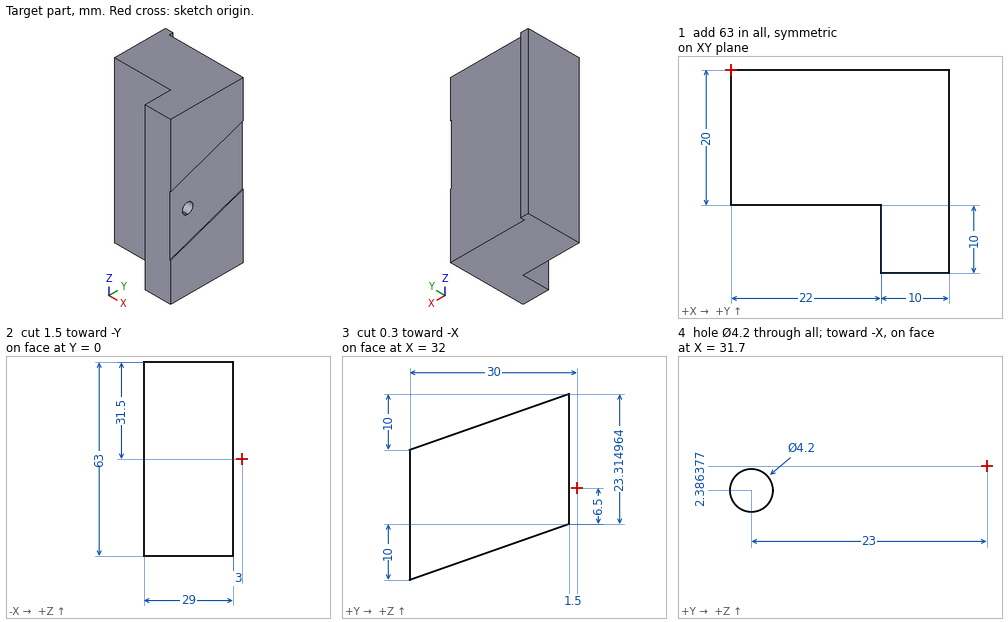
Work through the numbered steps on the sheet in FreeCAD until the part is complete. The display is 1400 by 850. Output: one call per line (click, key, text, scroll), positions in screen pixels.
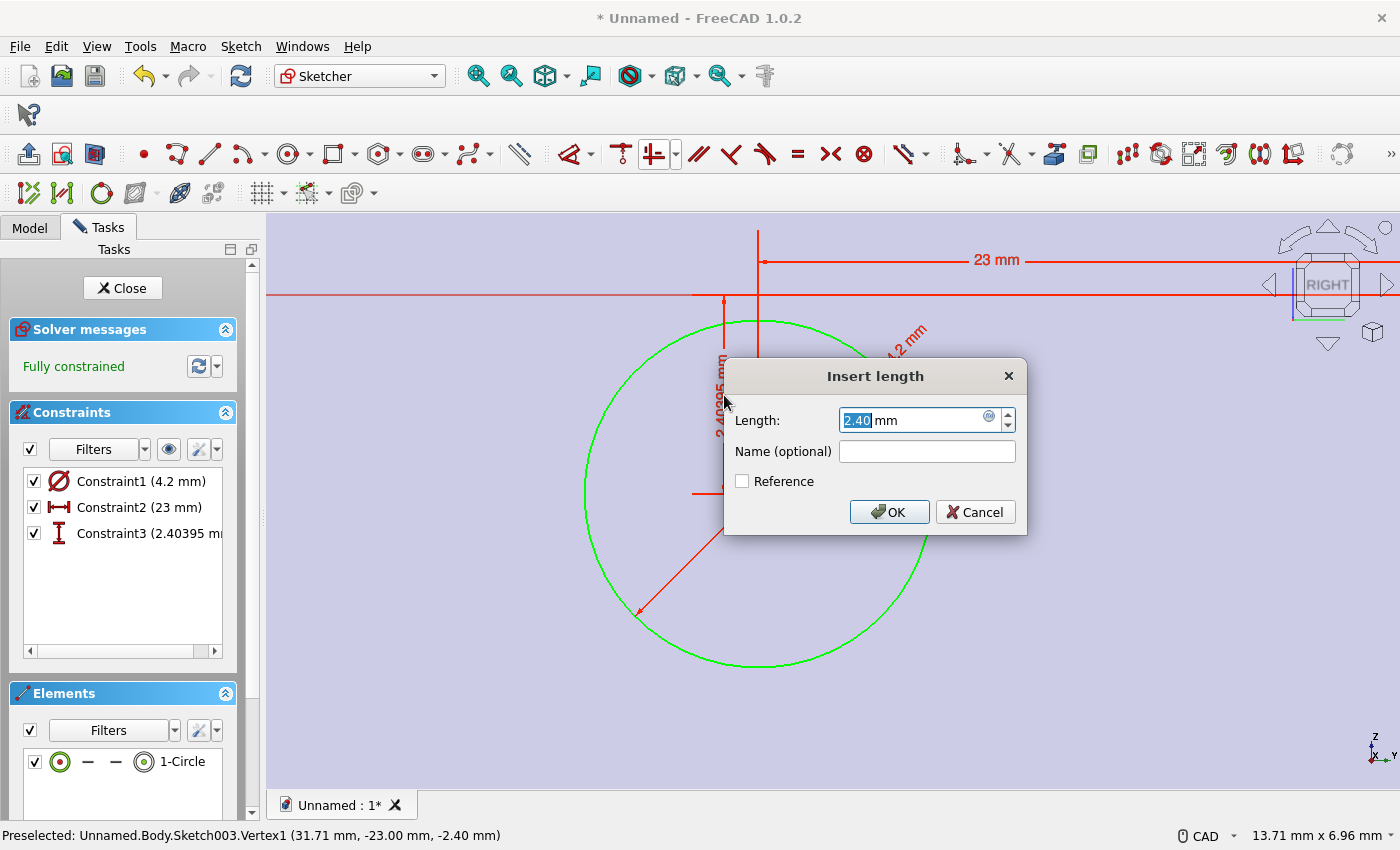
text(2.386377)
key(Return)
key(Escape)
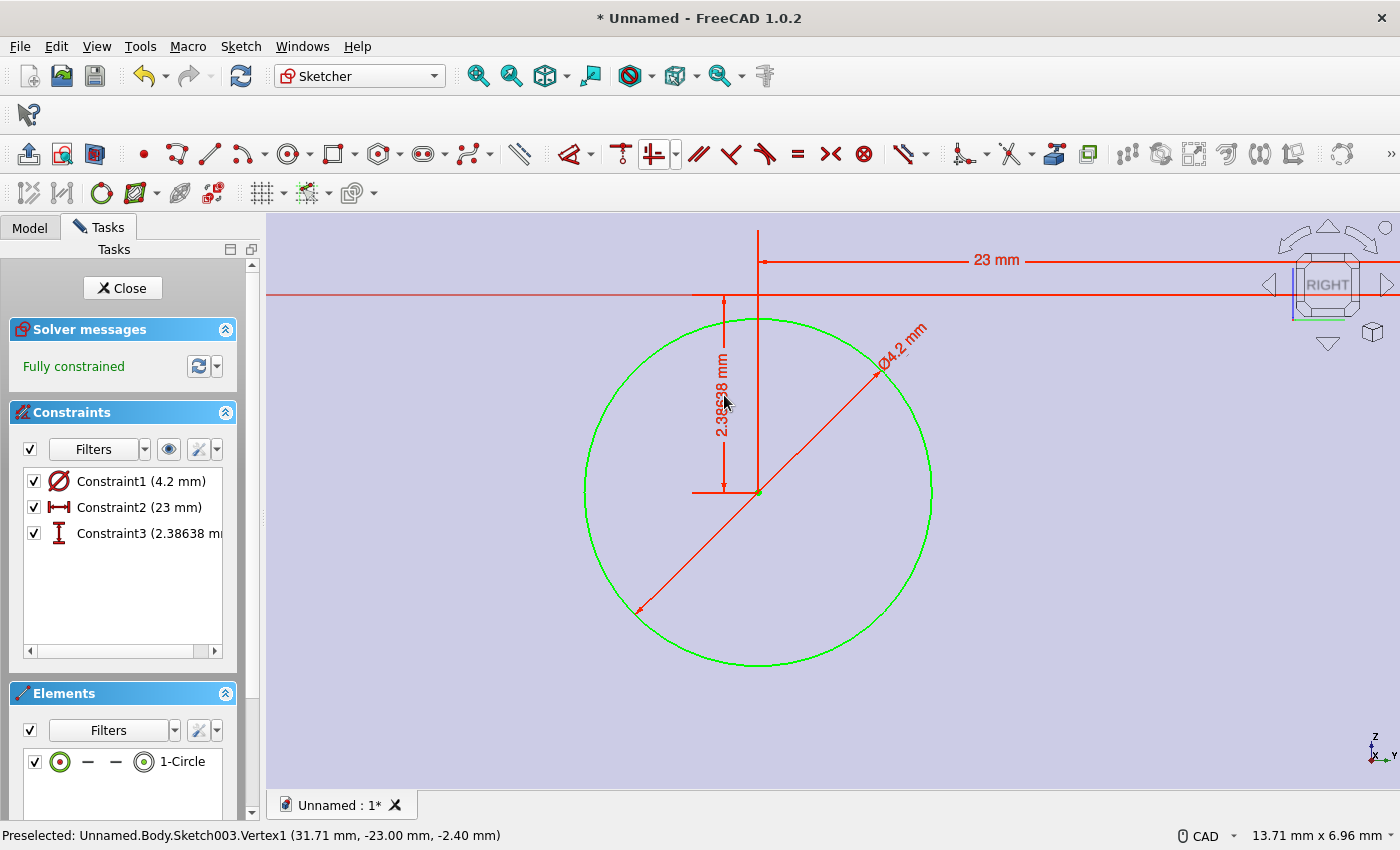
click(123, 288)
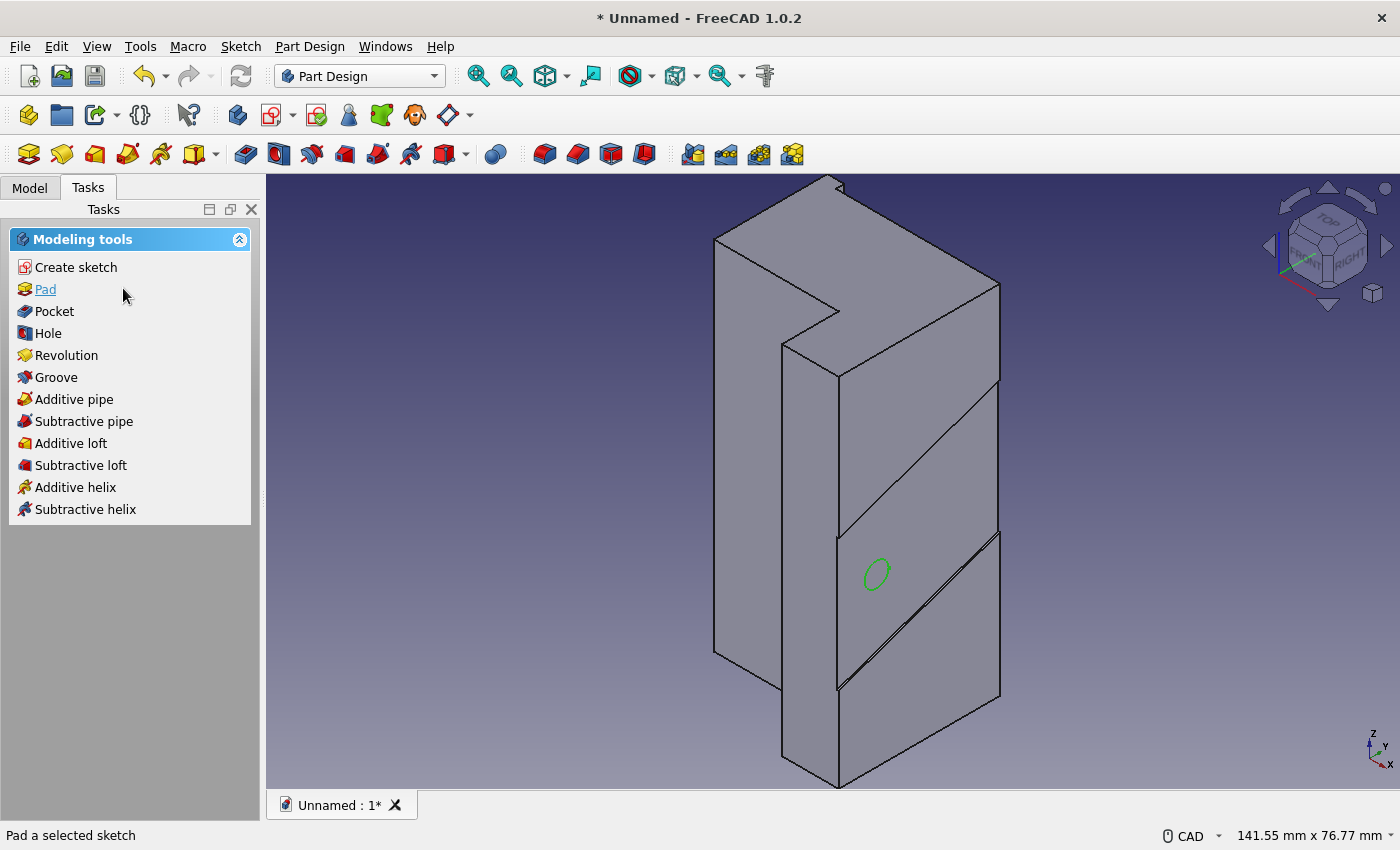
click(279, 154)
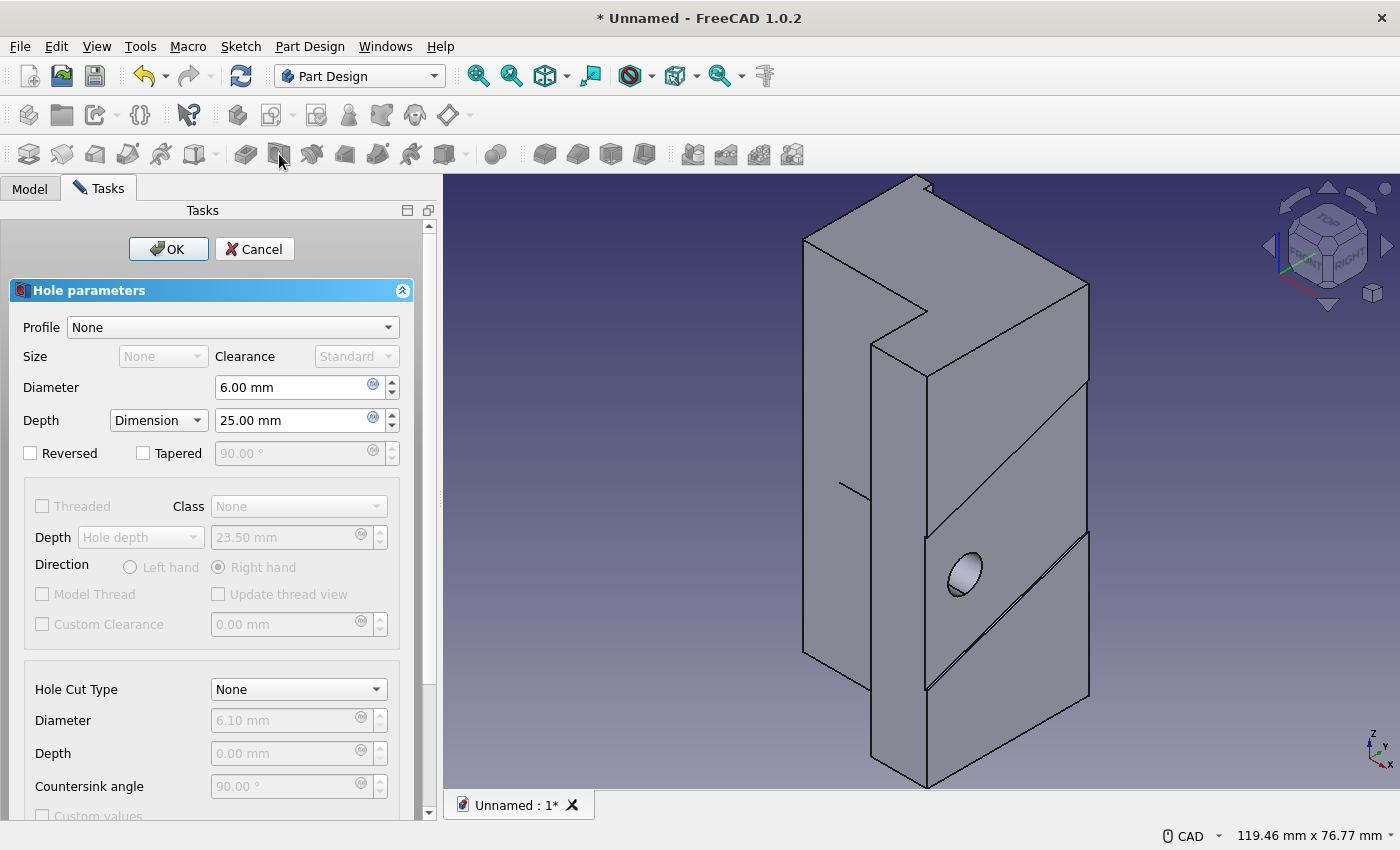
triple_click(300, 388)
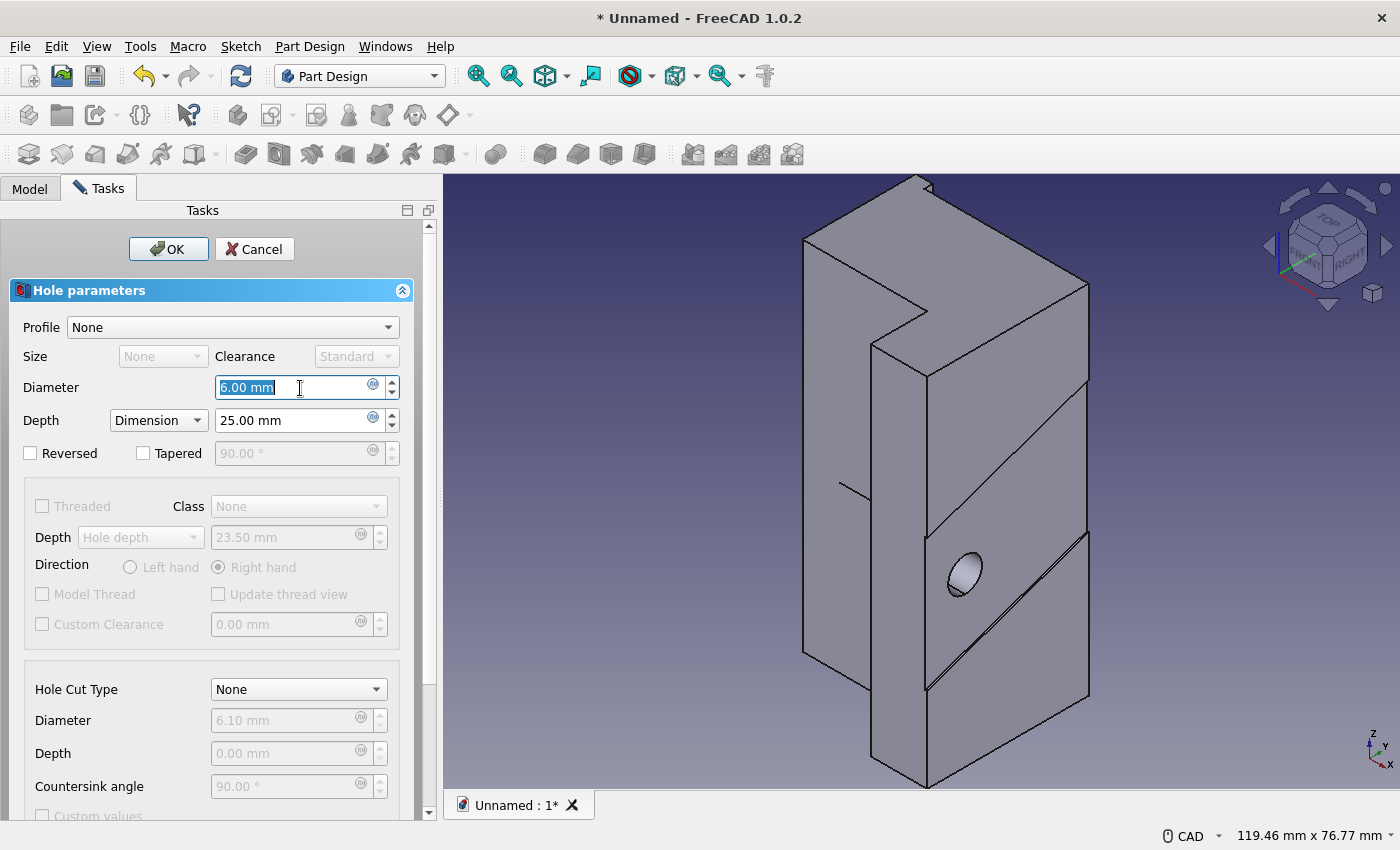
text(4.2)
key(Tab)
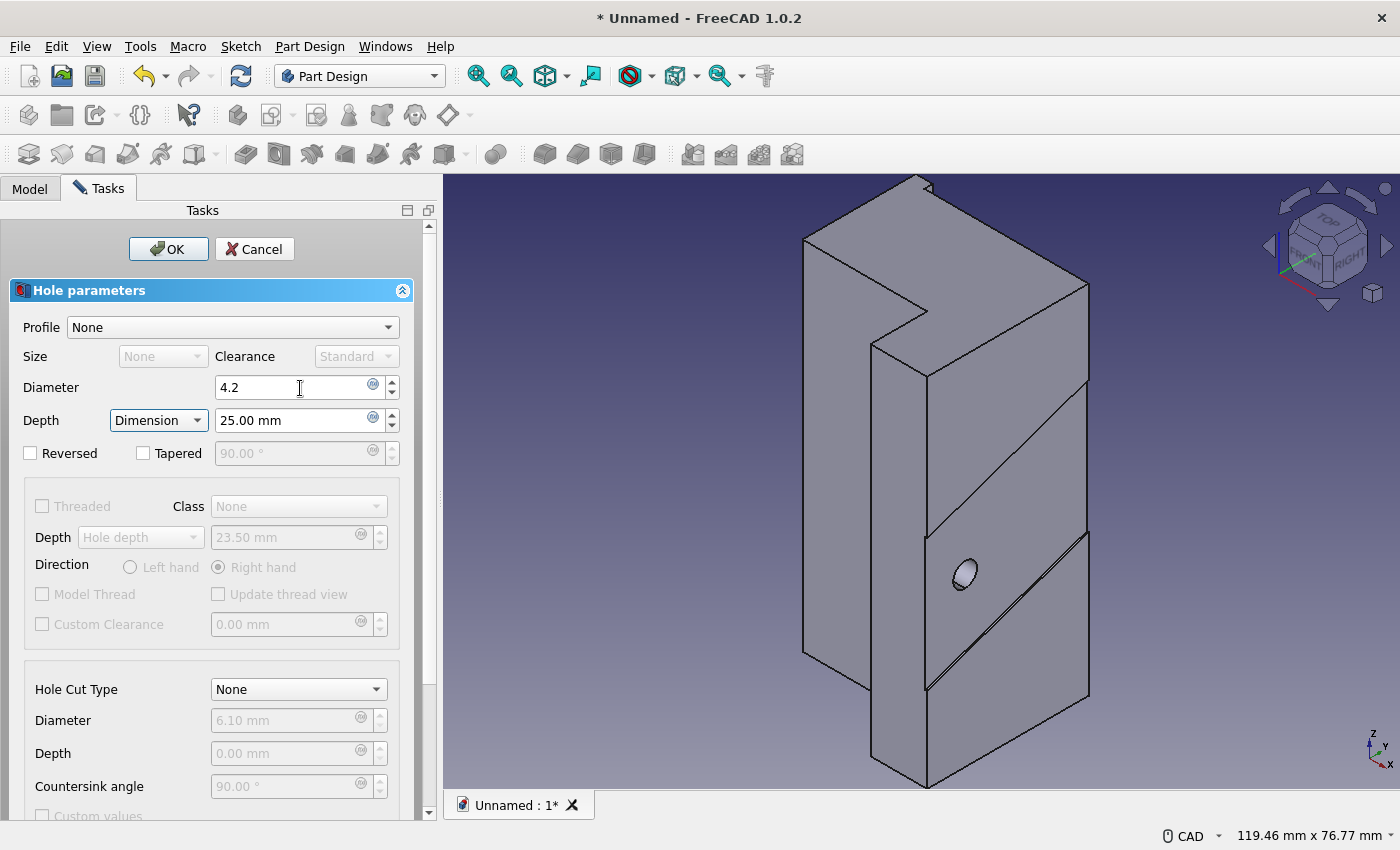
click(160, 420)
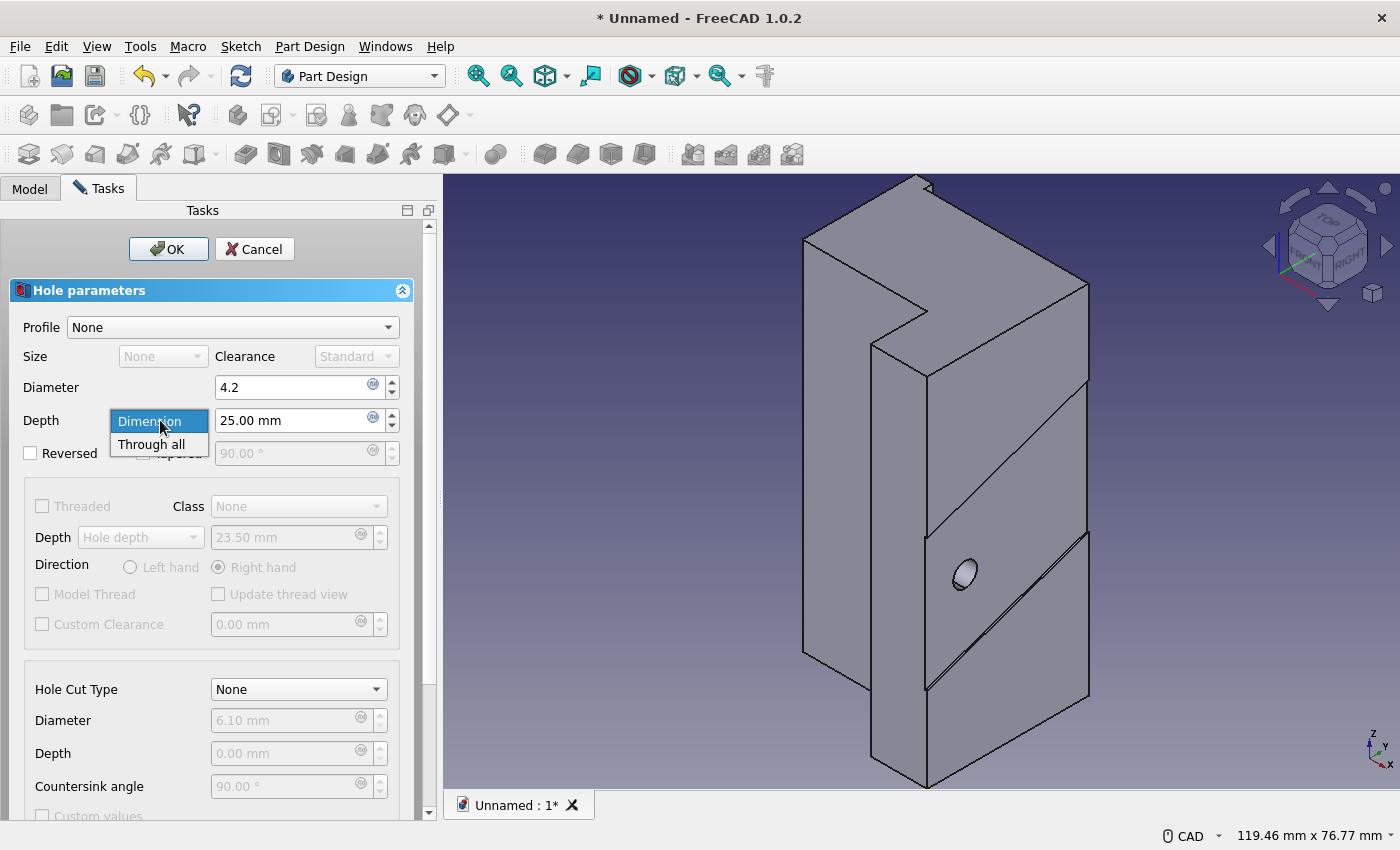
click(158, 444)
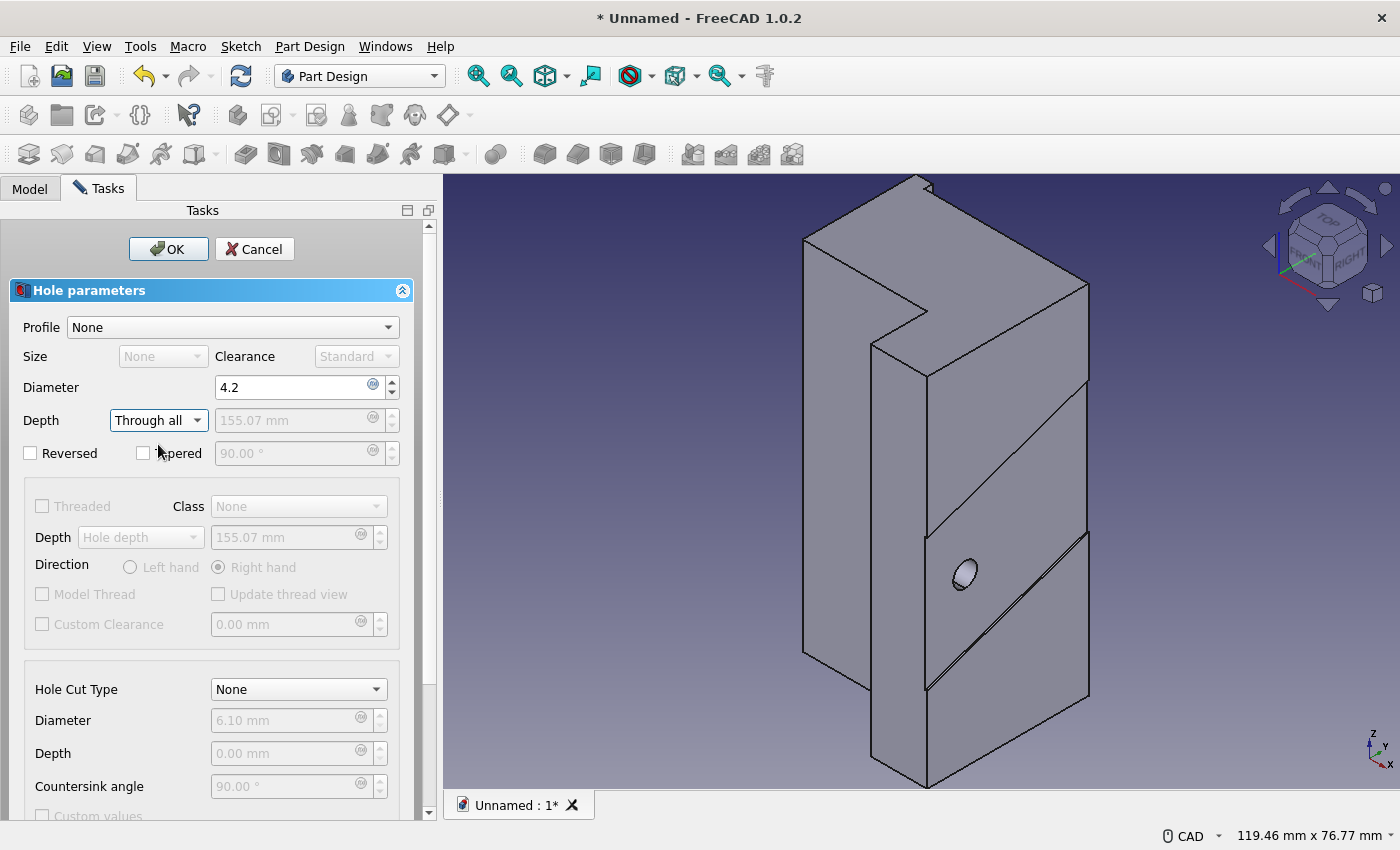
click(169, 249)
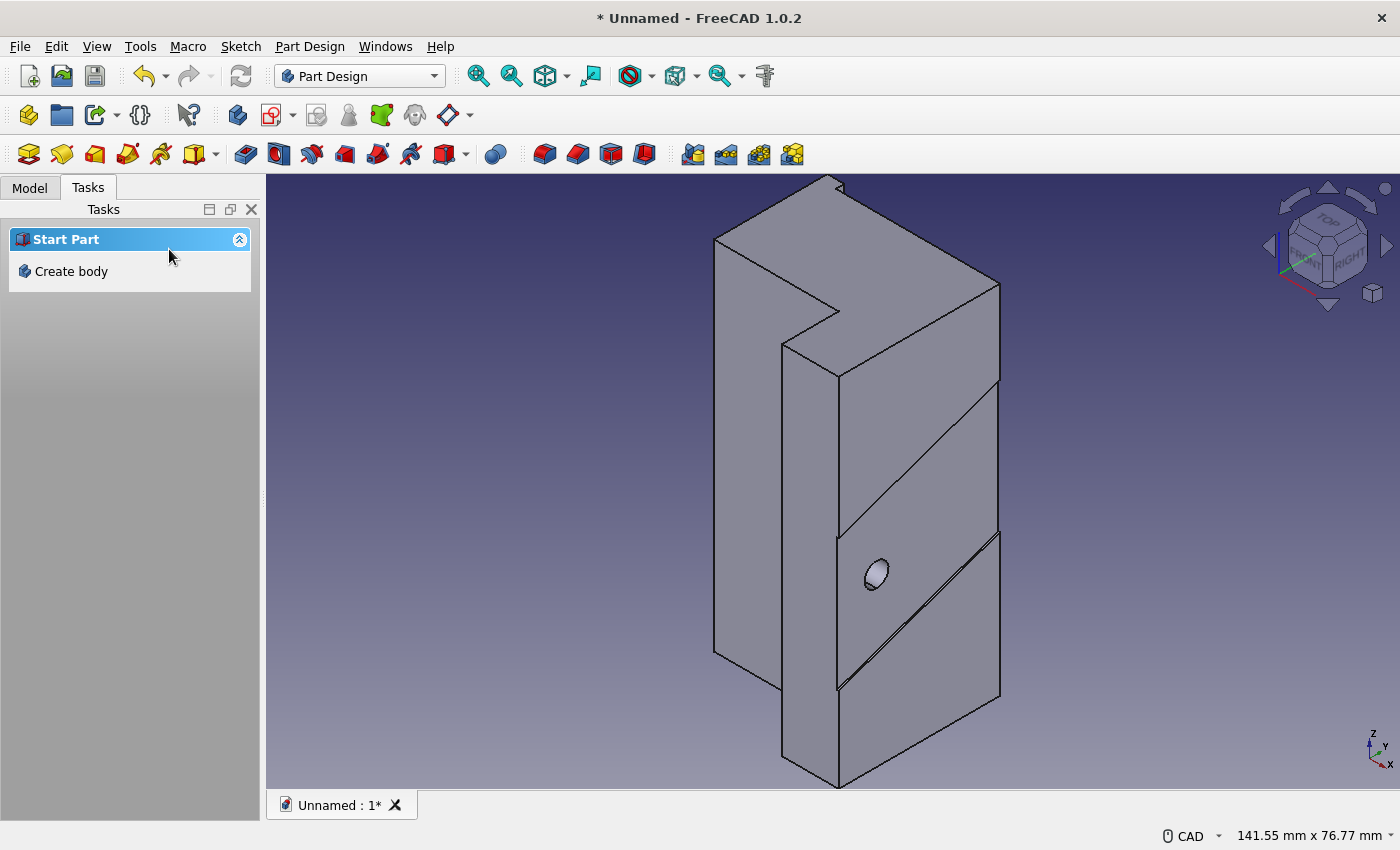
click(479, 76)